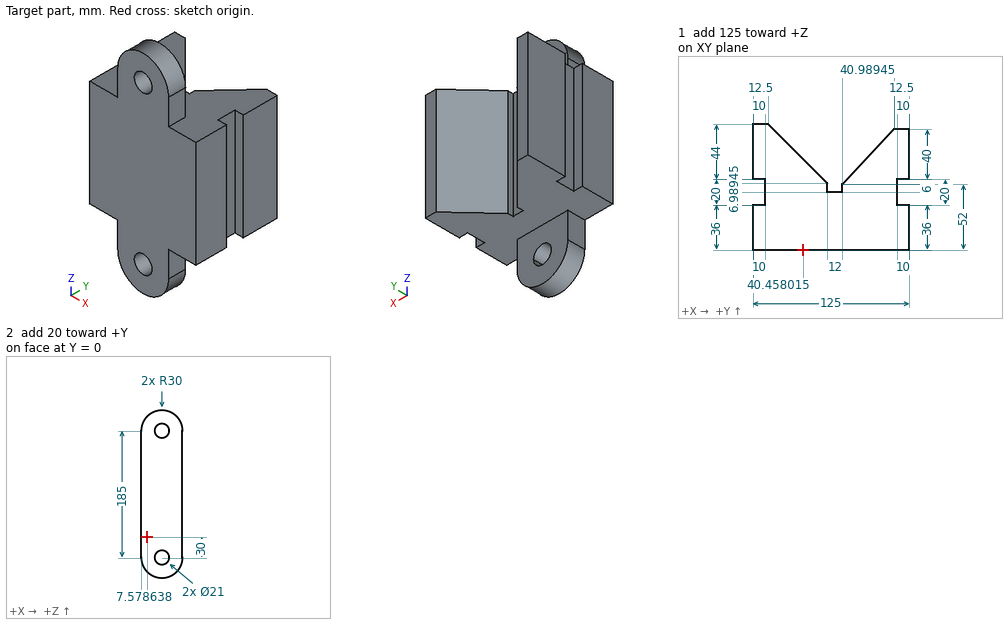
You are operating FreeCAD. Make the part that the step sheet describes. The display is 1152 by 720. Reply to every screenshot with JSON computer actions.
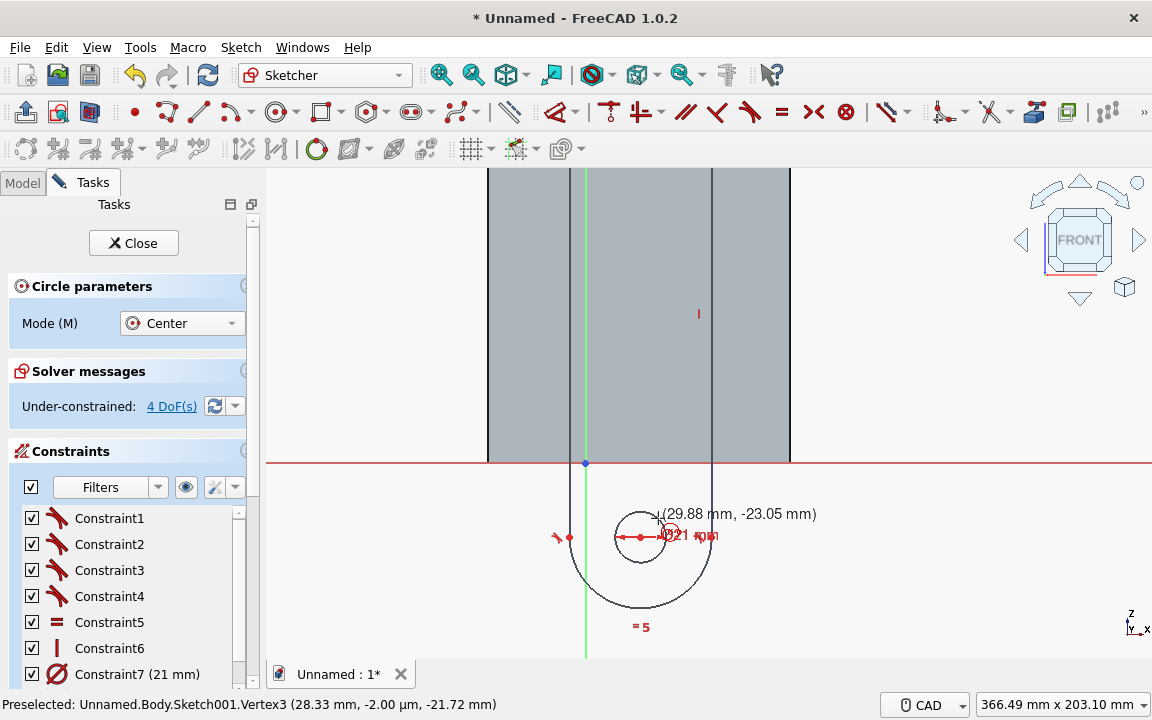
{"action": "scroll", "coordinate": [641, 537], "scroll_direction": "down", "scroll_amount": 3}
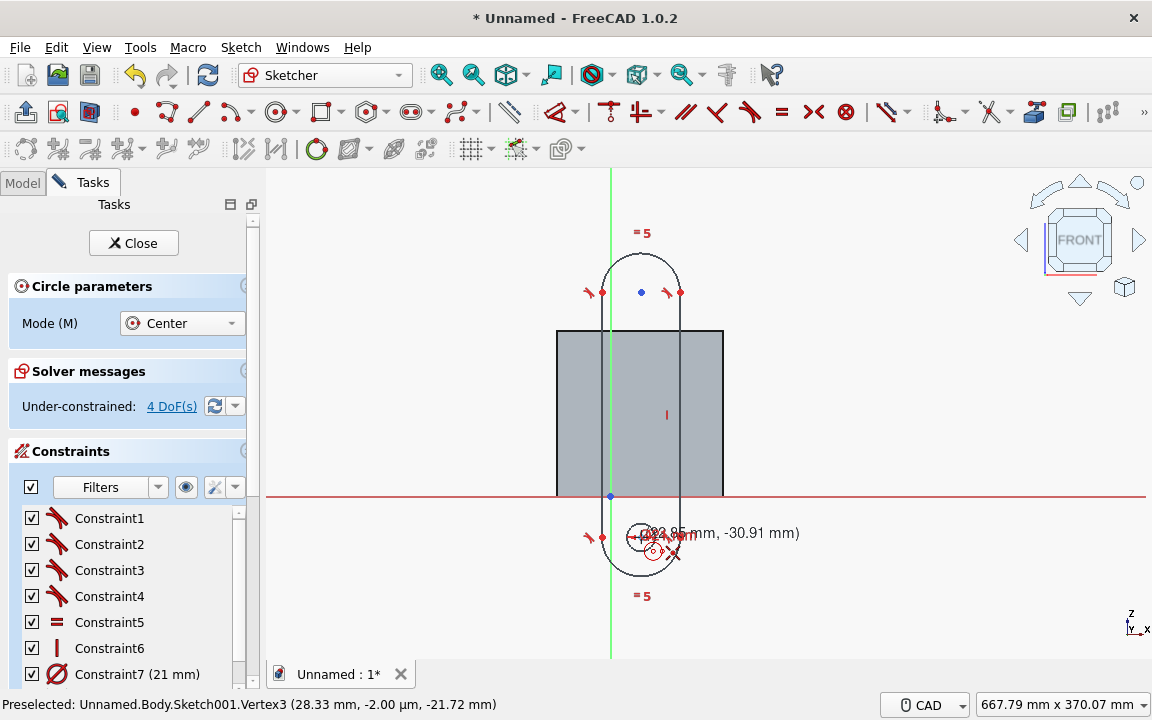
{"action": "scroll", "coordinate": [641, 291], "scroll_direction": "up", "scroll_amount": 3}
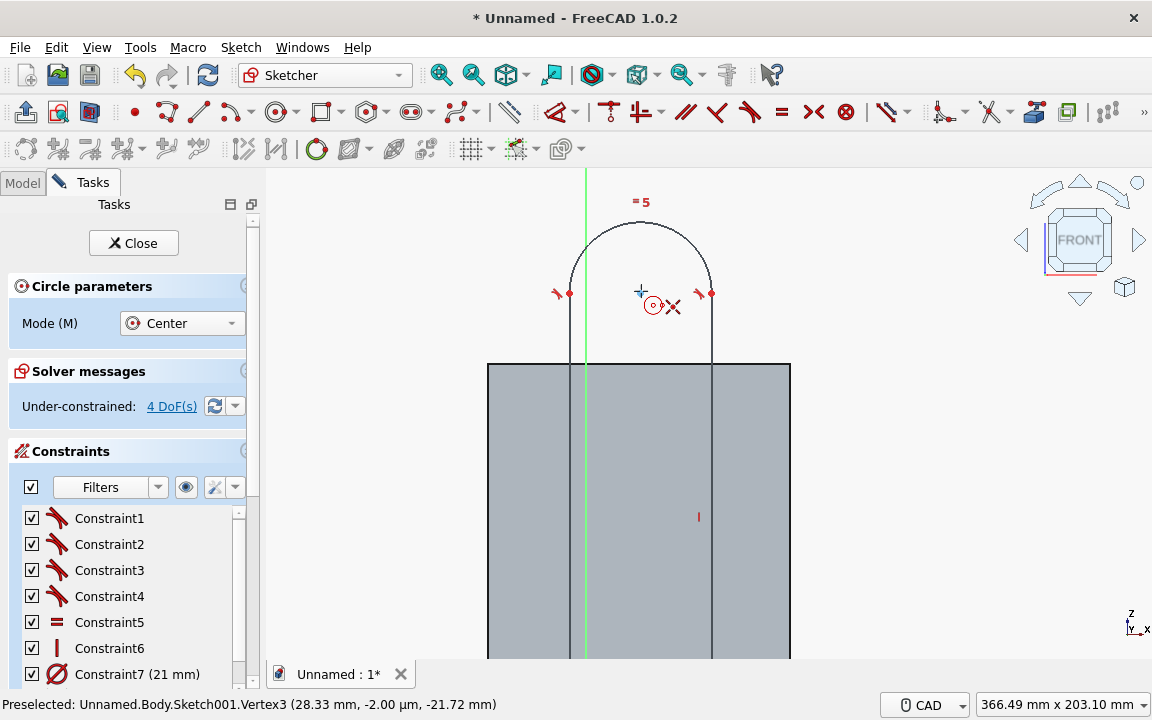
{"action": "left_click", "coordinate": [641, 293]}
{"action": "mouse_move", "coordinate": [658, 273]}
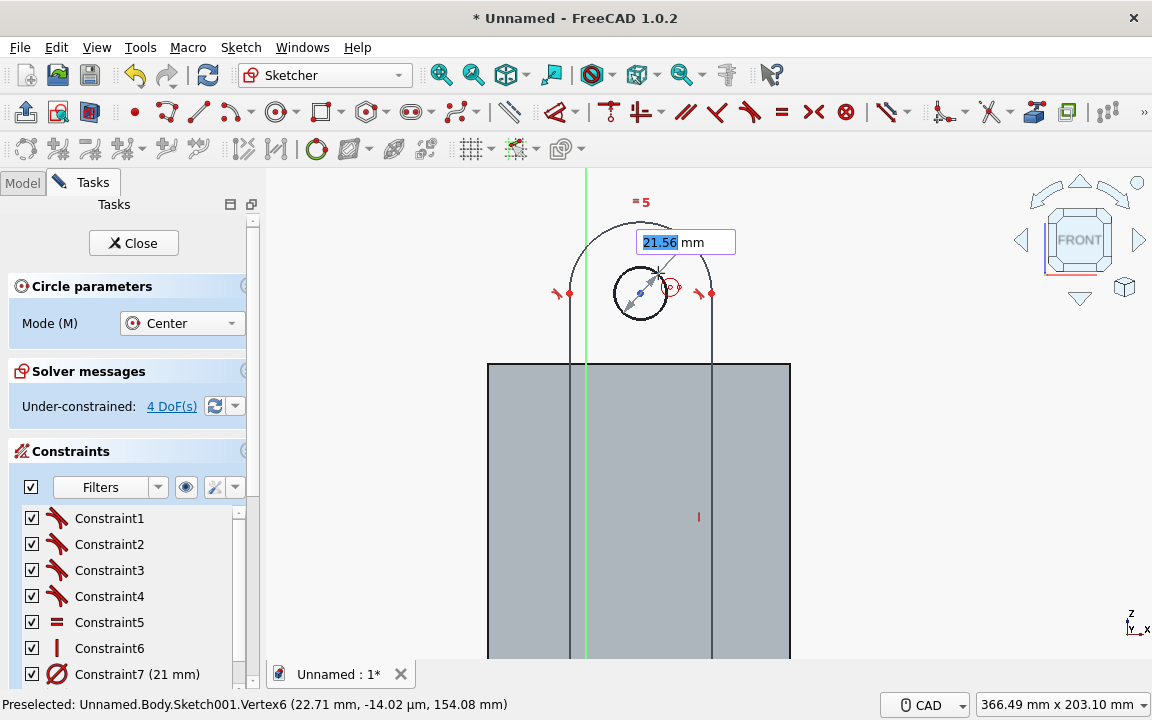
{"action": "type", "text": "21"}
{"action": "key", "text": "Return"}
{"action": "key", "text": "Escape"}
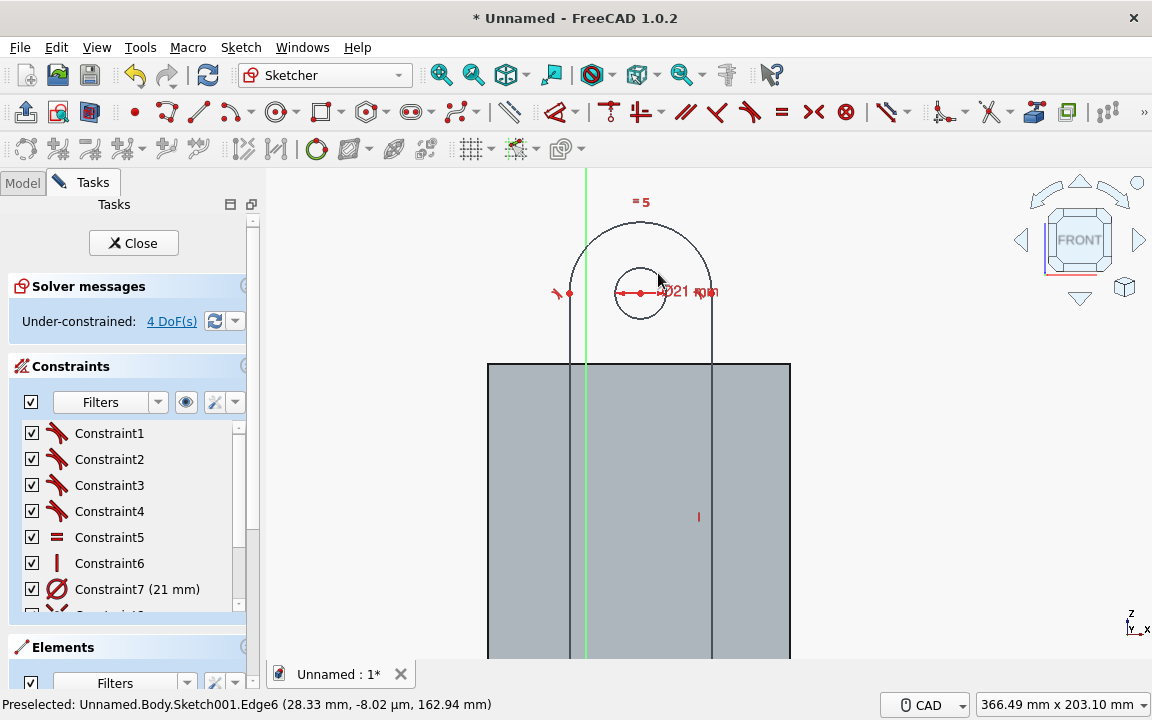
{"action": "key", "text": "d"}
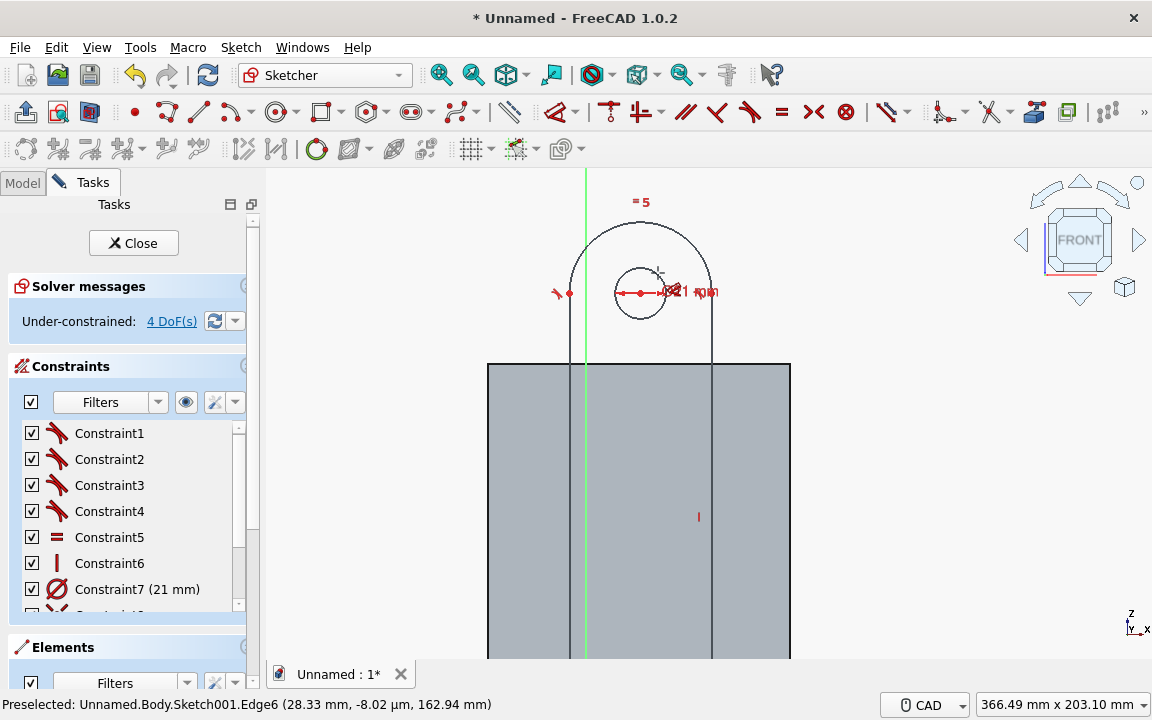
{"action": "scroll", "coordinate": [641, 290], "scroll_direction": "down", "scroll_amount": 3}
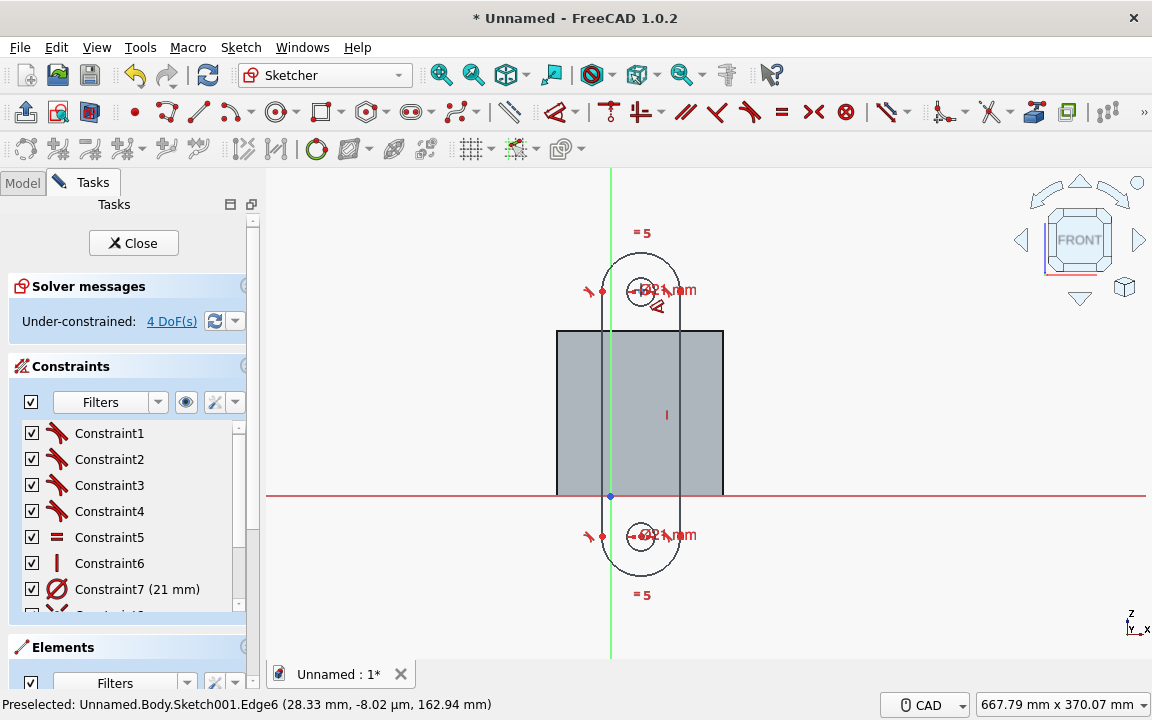
{"action": "scroll", "coordinate": [618, 569], "scroll_direction": "up", "scroll_amount": 4}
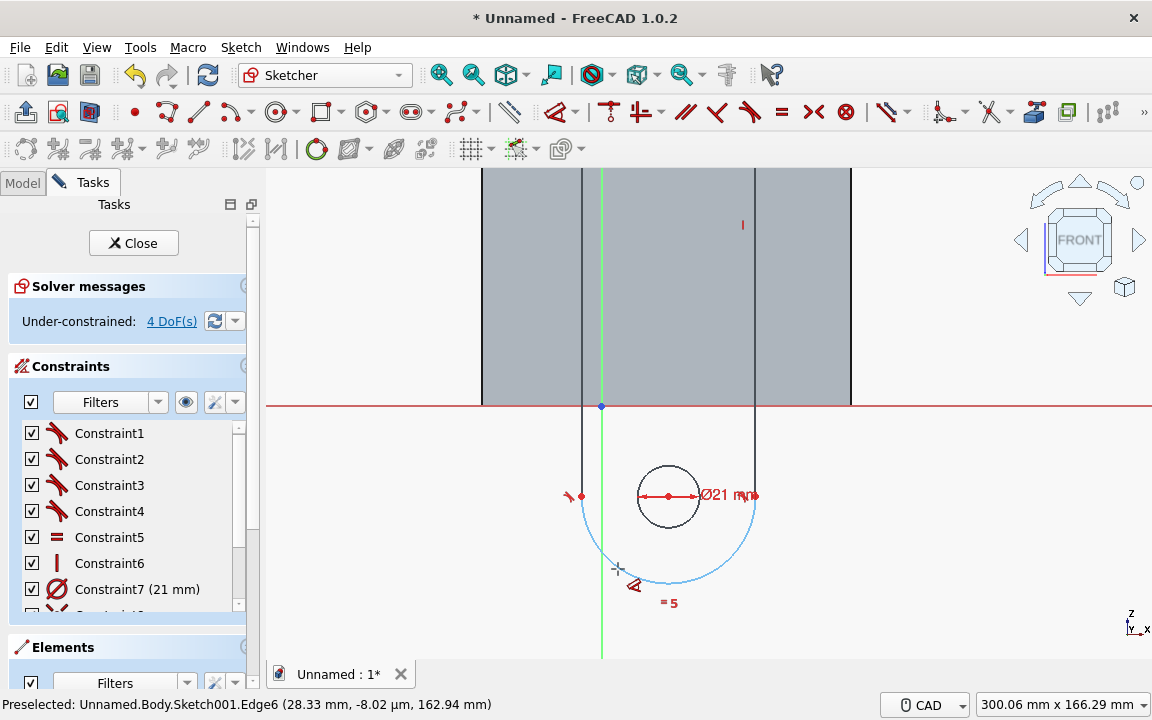
{"action": "left_click", "coordinate": [618, 567]}
{"action": "left_click", "coordinate": [562, 548]}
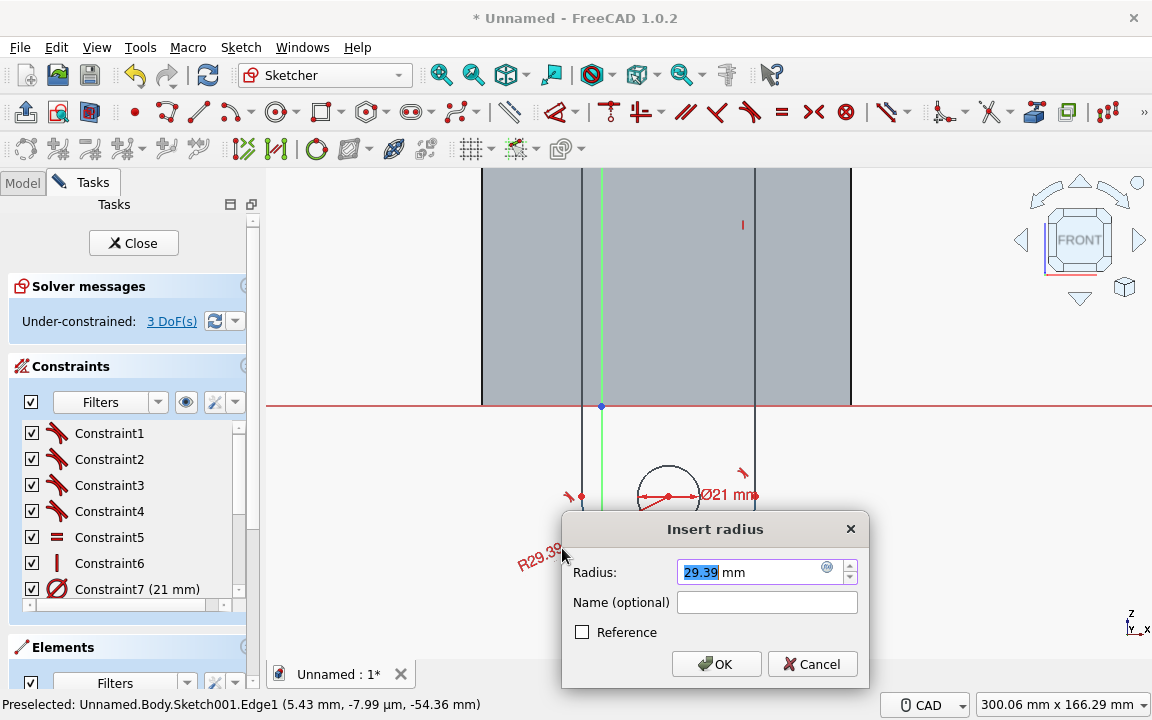
{"action": "type", "text": "30"}
{"action": "key", "text": "Return"}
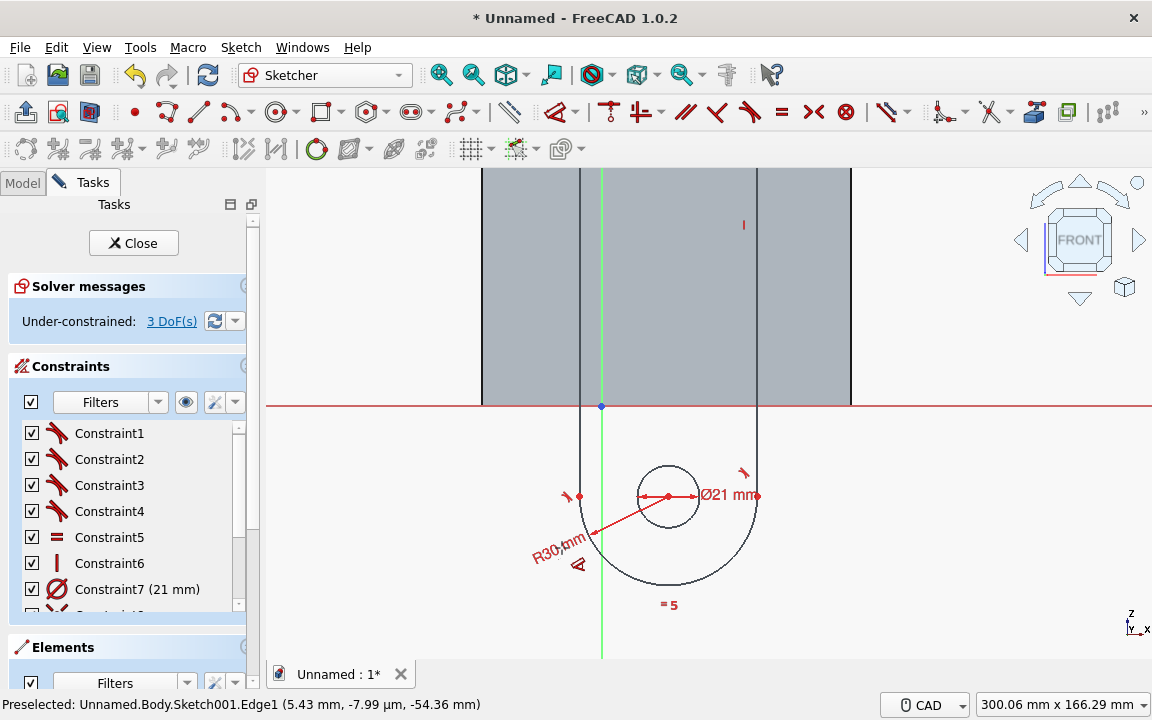
{"action": "left_click", "coordinate": [668, 497]}
{"action": "left_click", "coordinate": [702, 452]}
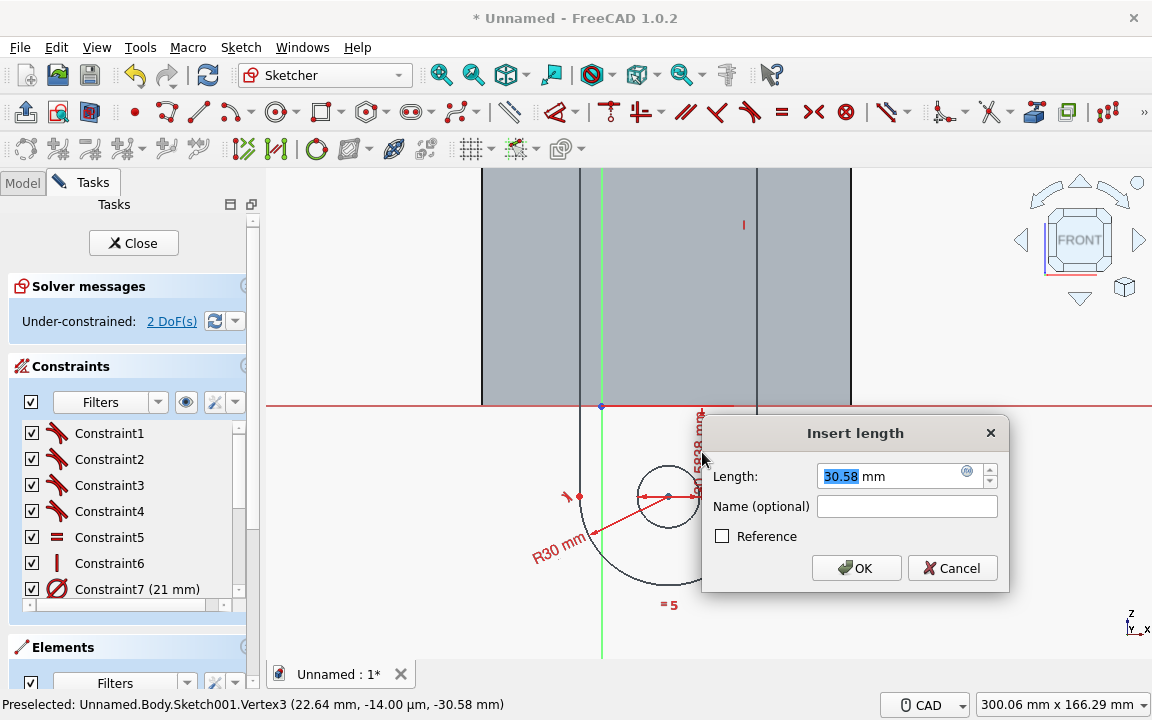
{"action": "type", "text": "30"}
{"action": "key", "text": "Return"}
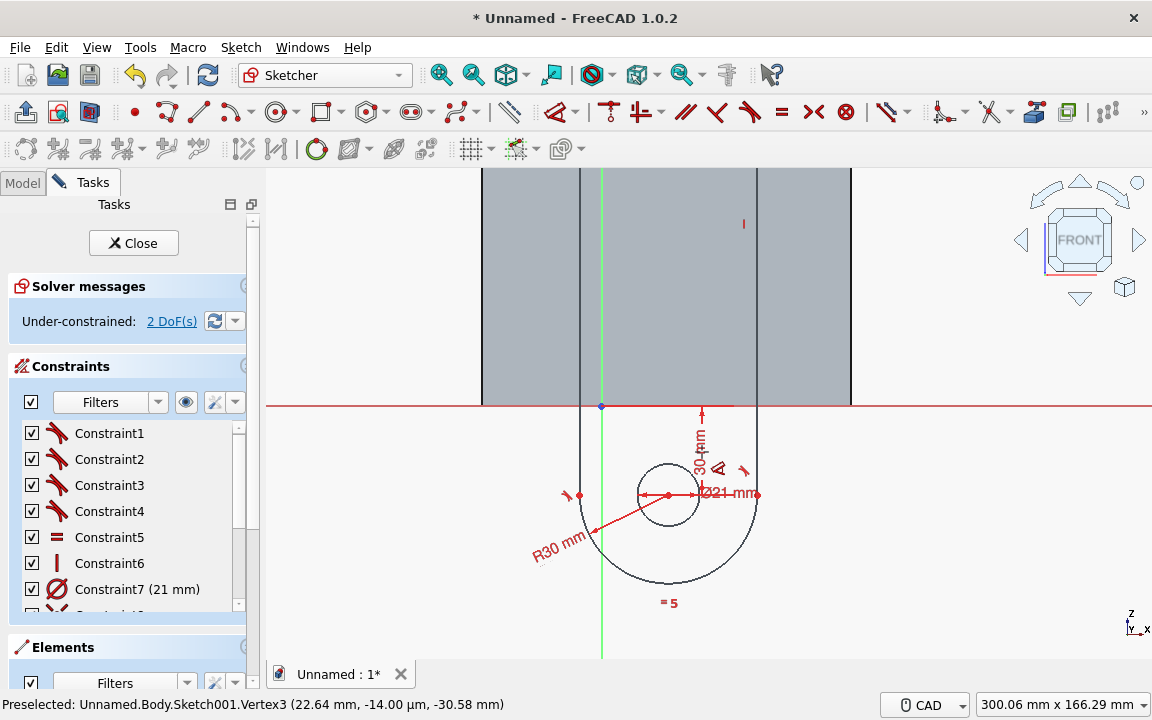
{"action": "left_click", "coordinate": [580, 332]}
{"action": "left_click", "coordinate": [546, 346]}